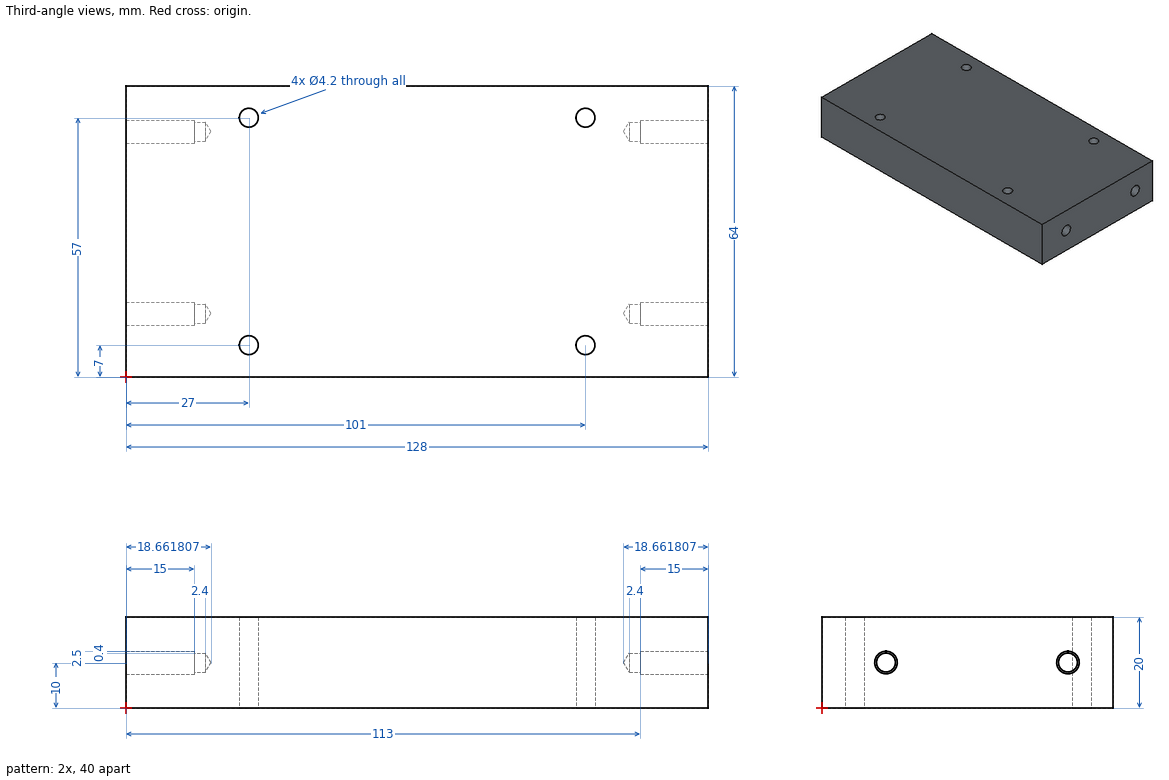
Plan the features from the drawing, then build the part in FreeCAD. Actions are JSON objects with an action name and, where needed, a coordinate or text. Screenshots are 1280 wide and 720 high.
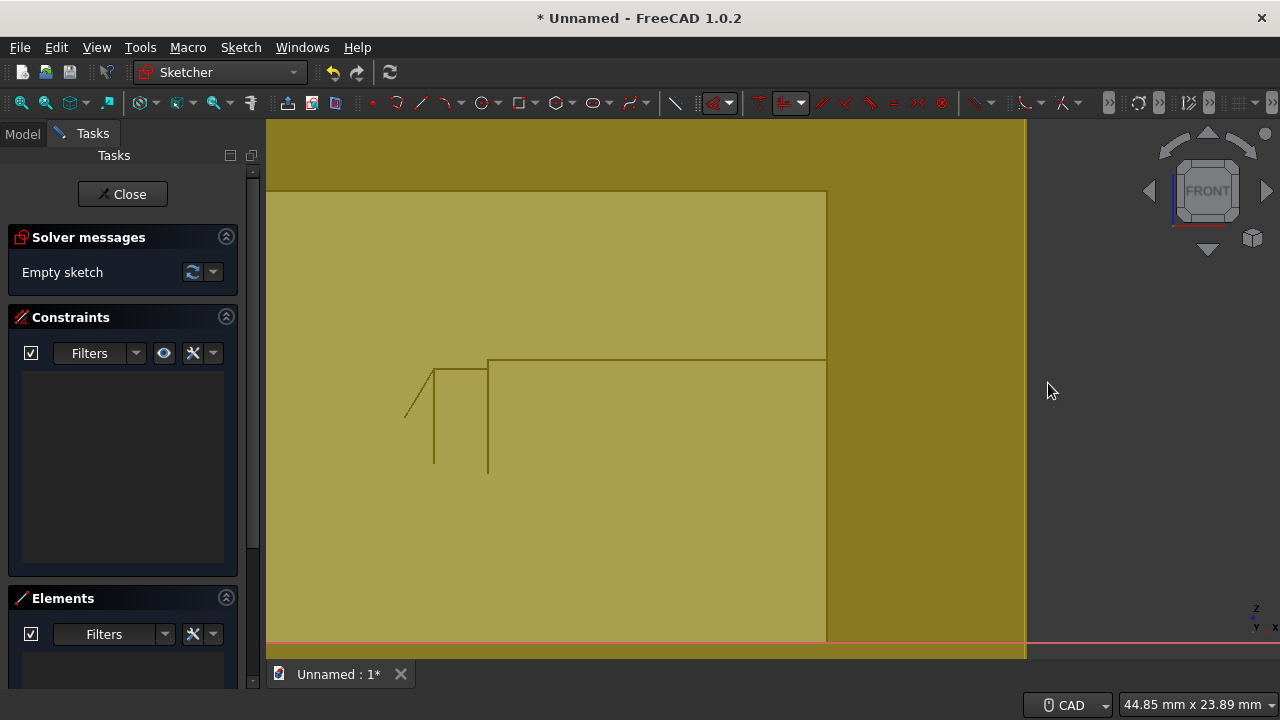
{"action": "left_click", "coordinate": [398, 104]}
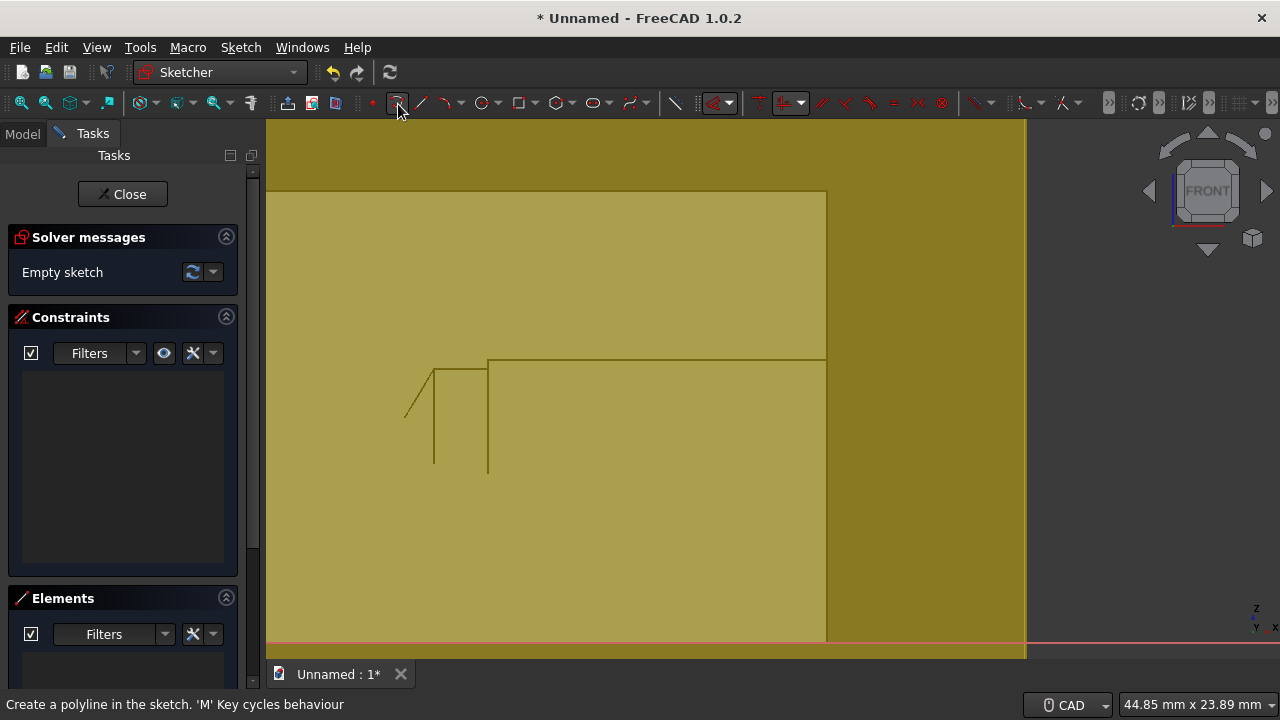
{"action": "left_click", "coordinate": [405, 417]}
{"action": "left_click", "coordinate": [434, 369]}
{"action": "left_click", "coordinate": [488, 369]}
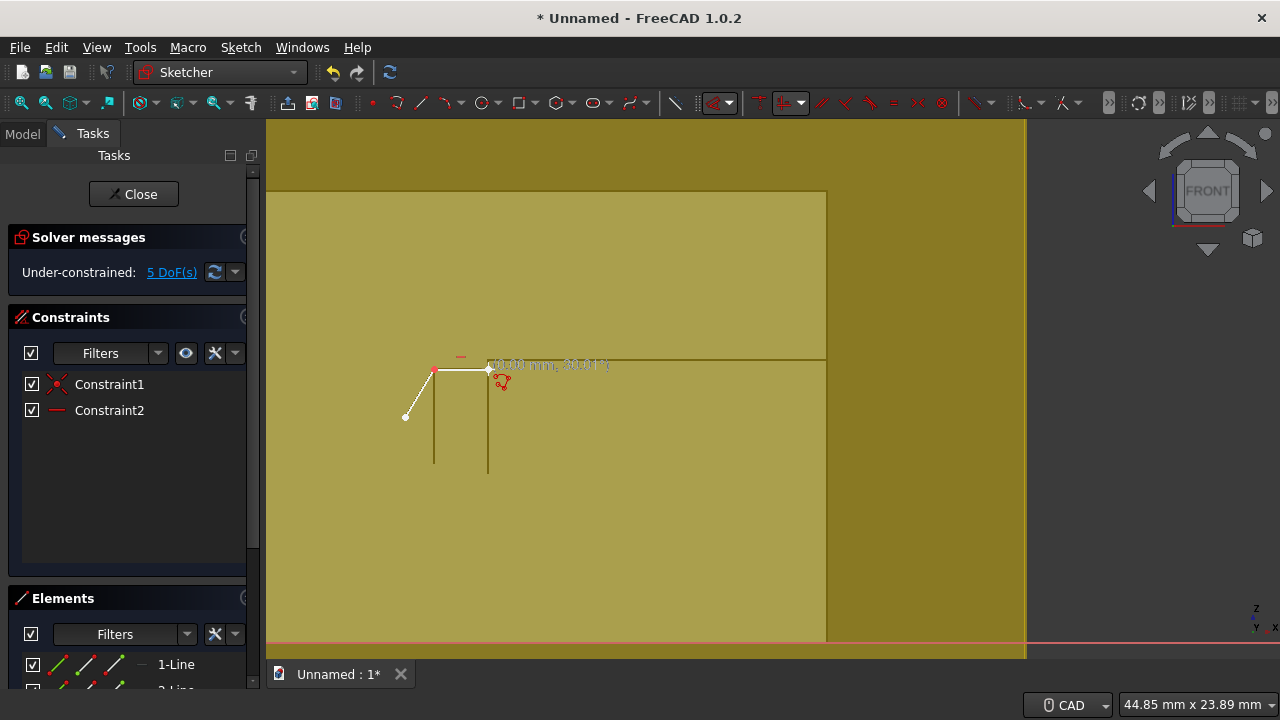
{"action": "scroll", "coordinate": [488, 360], "scroll_direction": "up", "scroll_amount": 3}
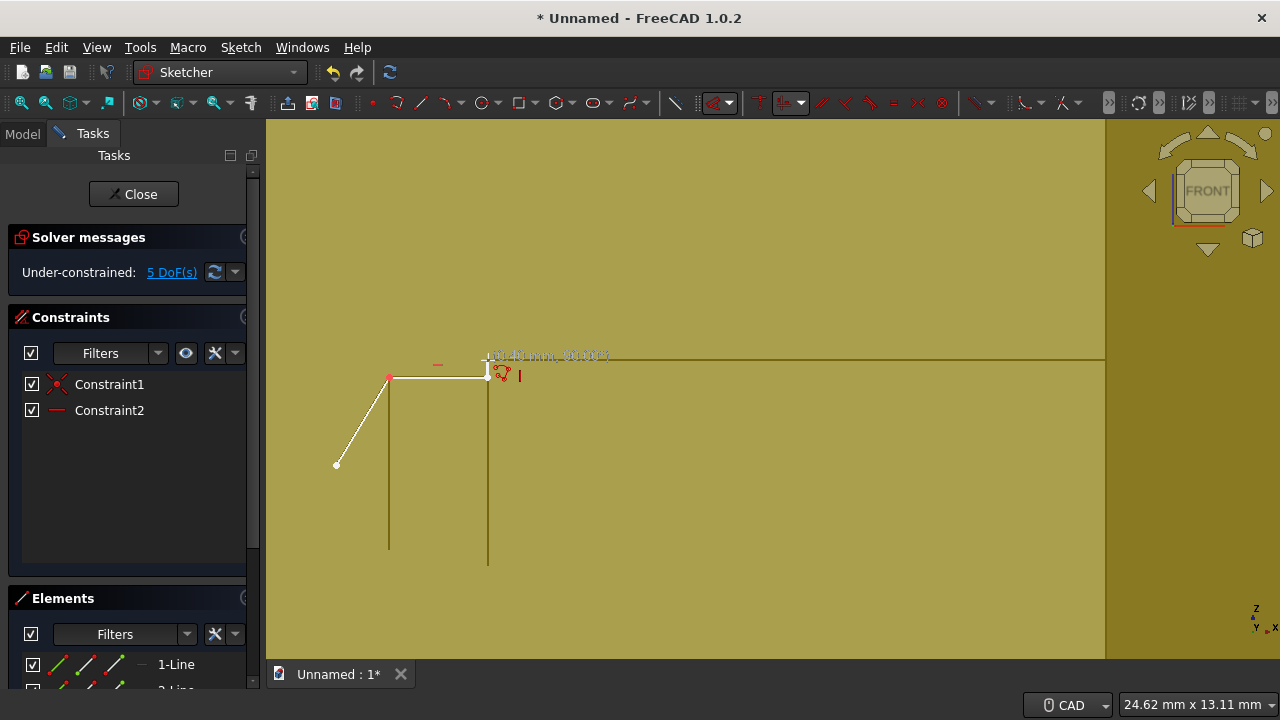
{"action": "left_click", "coordinate": [488, 360]}
{"action": "left_click", "coordinate": [1106, 360]}
{"action": "left_click", "coordinate": [1106, 463]}
{"action": "left_click", "coordinate": [337, 465]}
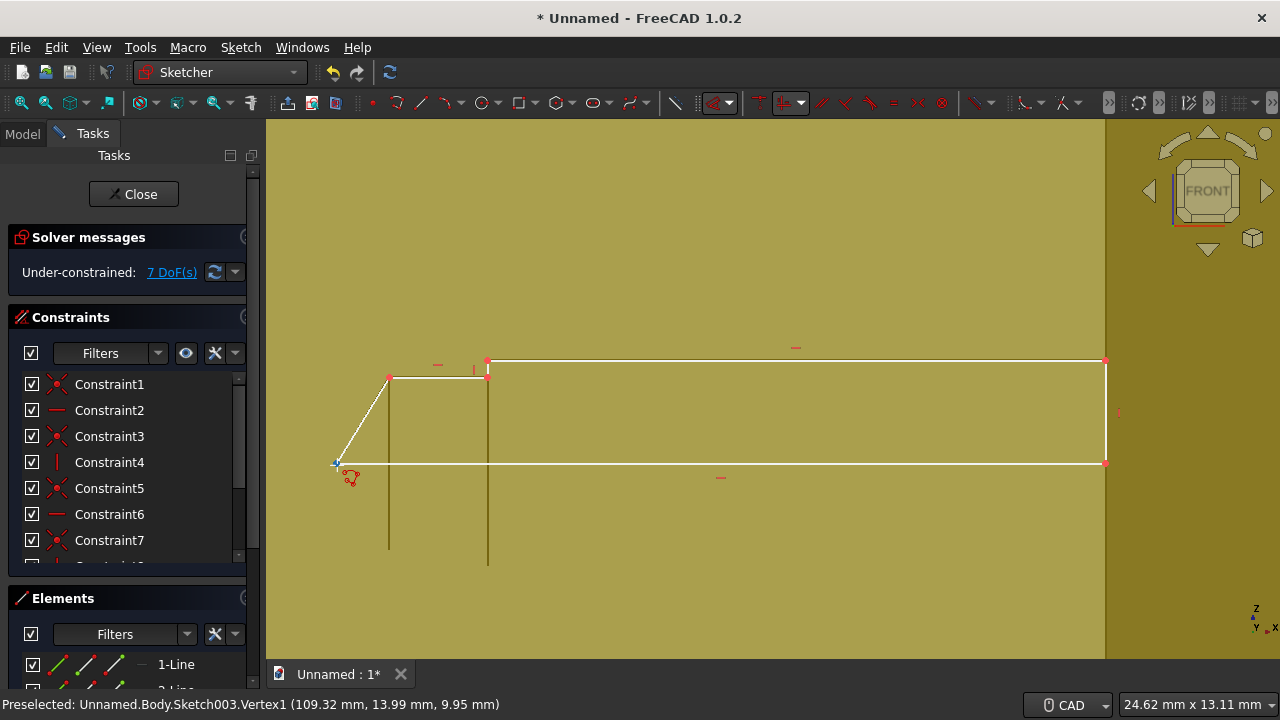
{"action": "left_click", "coordinate": [422, 104]}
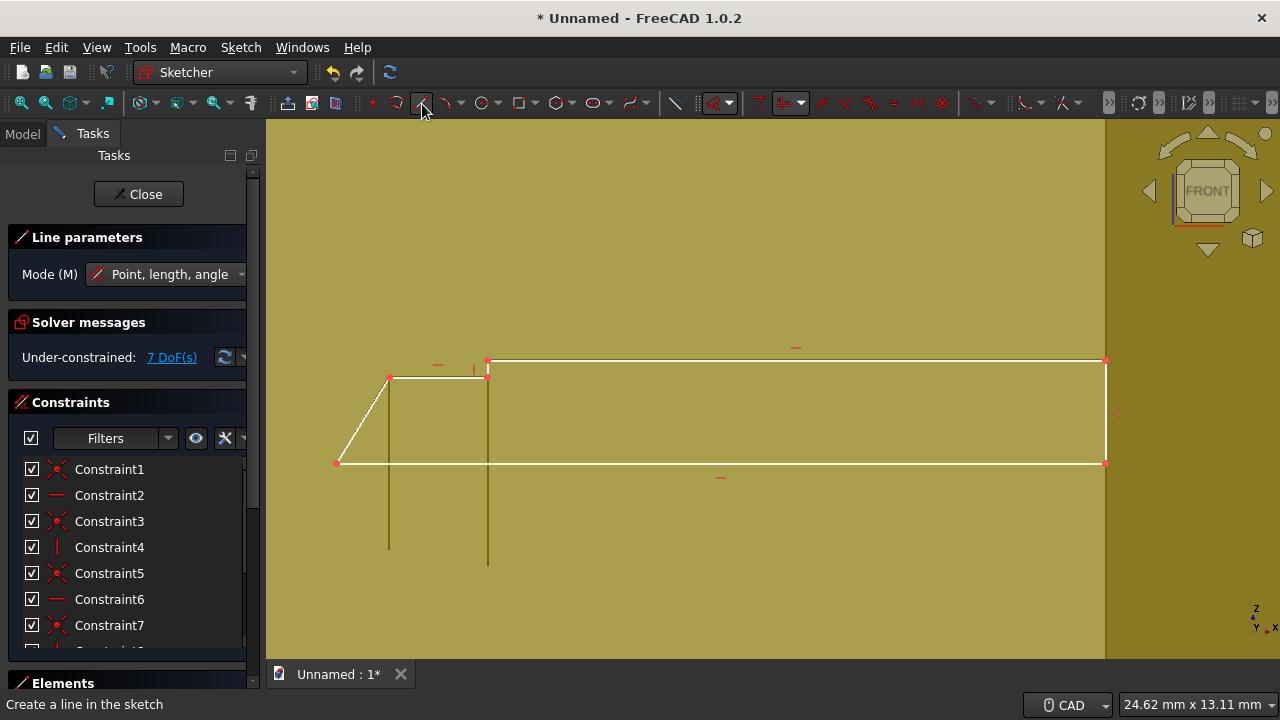
{"action": "scroll", "coordinate": [496, 361], "scroll_direction": "down", "scroll_amount": 3}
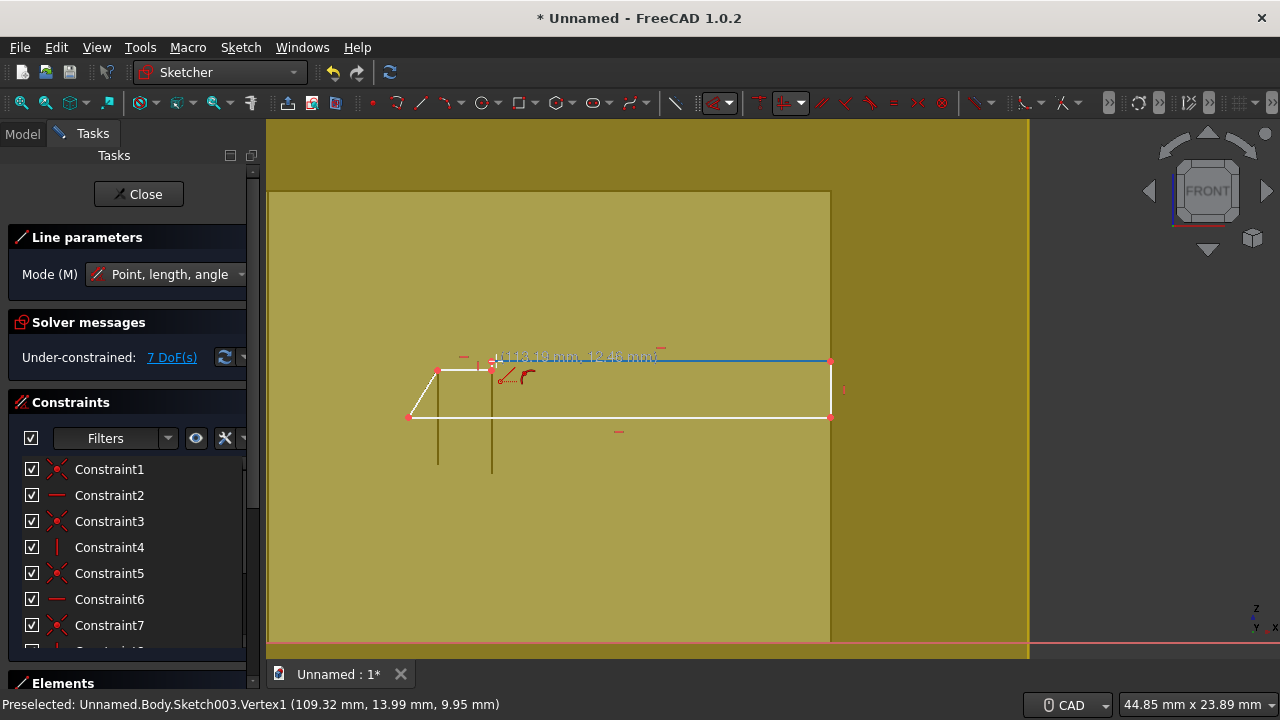
{"action": "left_click", "coordinate": [873, 417]}
{"action": "left_click", "coordinate": [1000, 417]}
{"action": "key", "text": "Escape"}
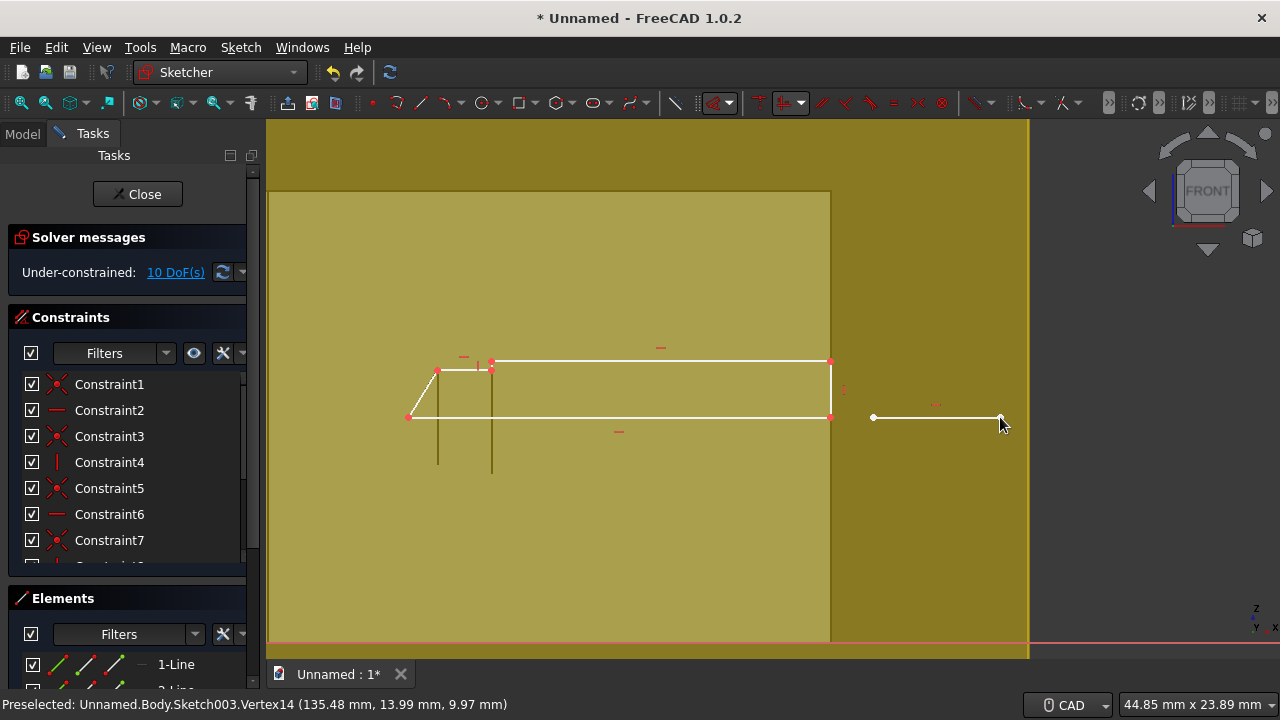
{"action": "left_click", "coordinate": [911, 418]}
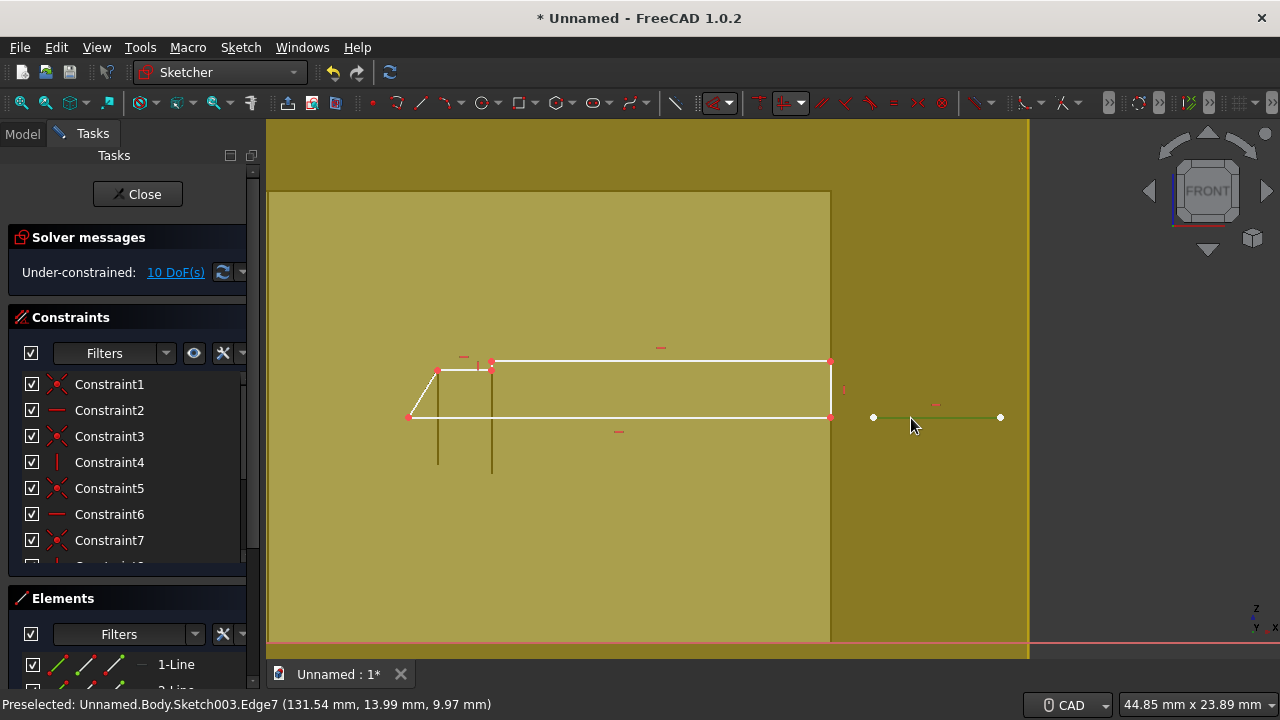
{"action": "left_click", "coordinate": [676, 104]}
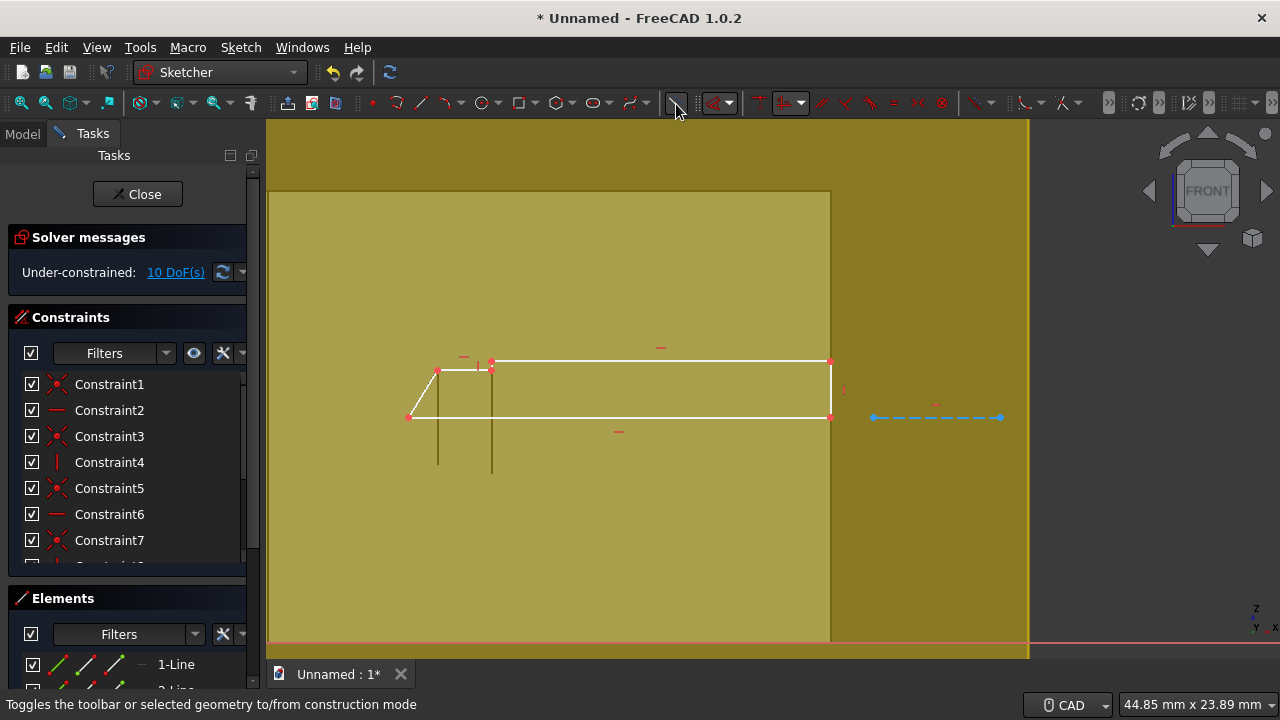
{"action": "left_click", "coordinate": [593, 361]}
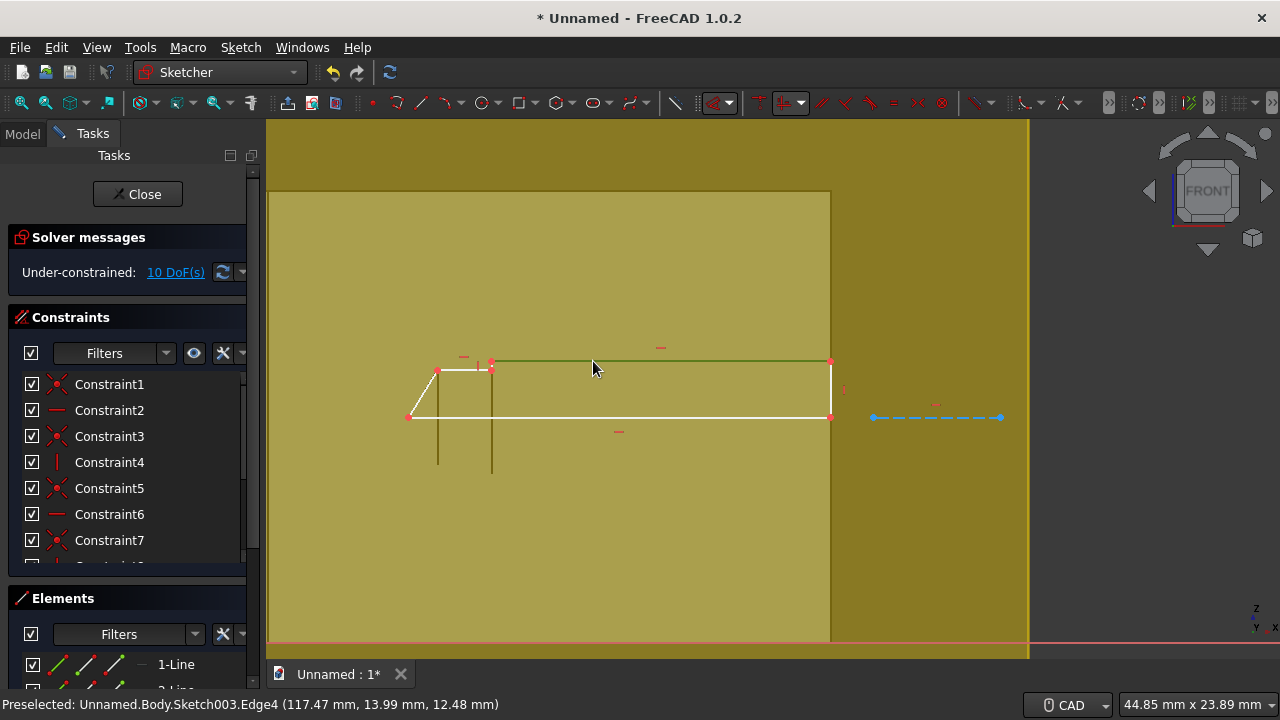
{"action": "key", "text": "l"}